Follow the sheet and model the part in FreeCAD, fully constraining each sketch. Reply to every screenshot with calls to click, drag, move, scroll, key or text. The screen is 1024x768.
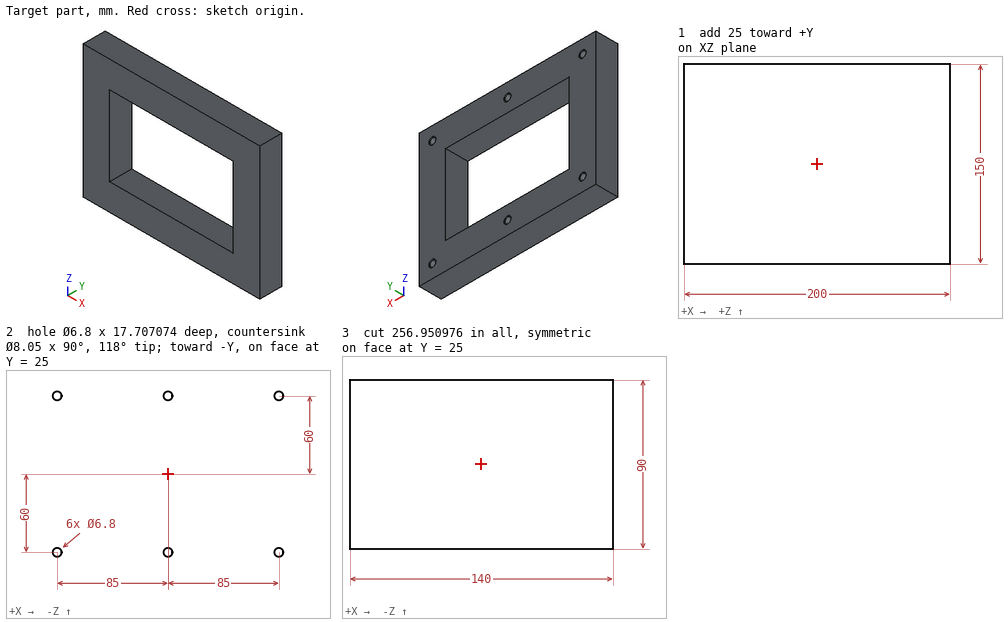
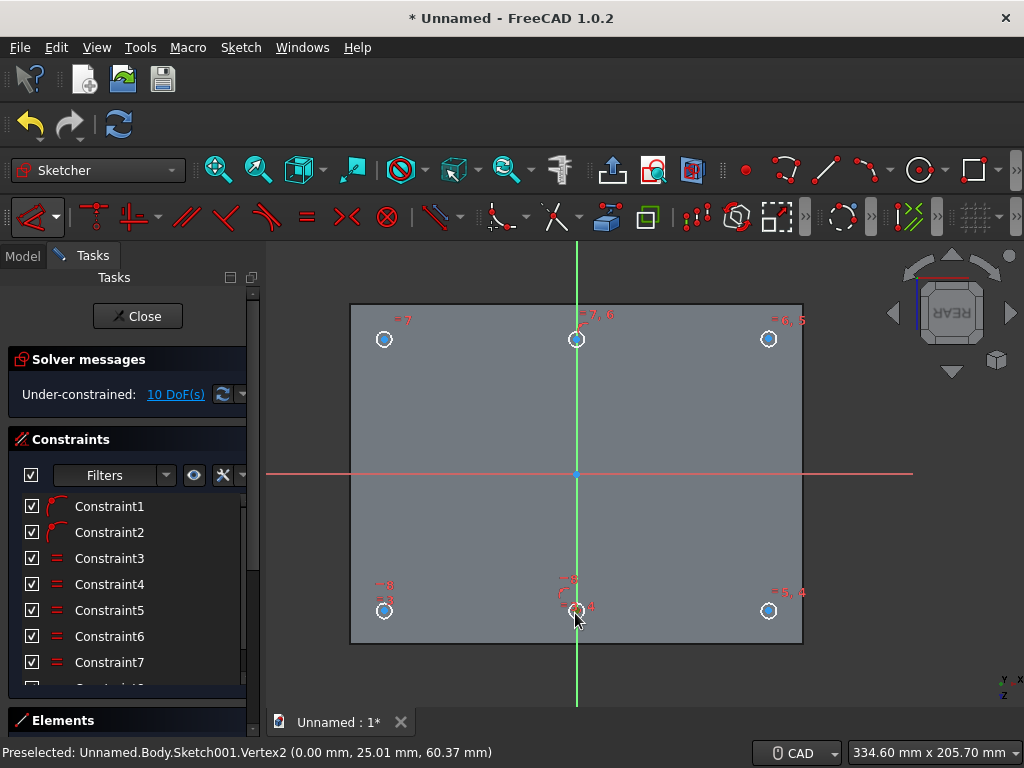
click(769, 611)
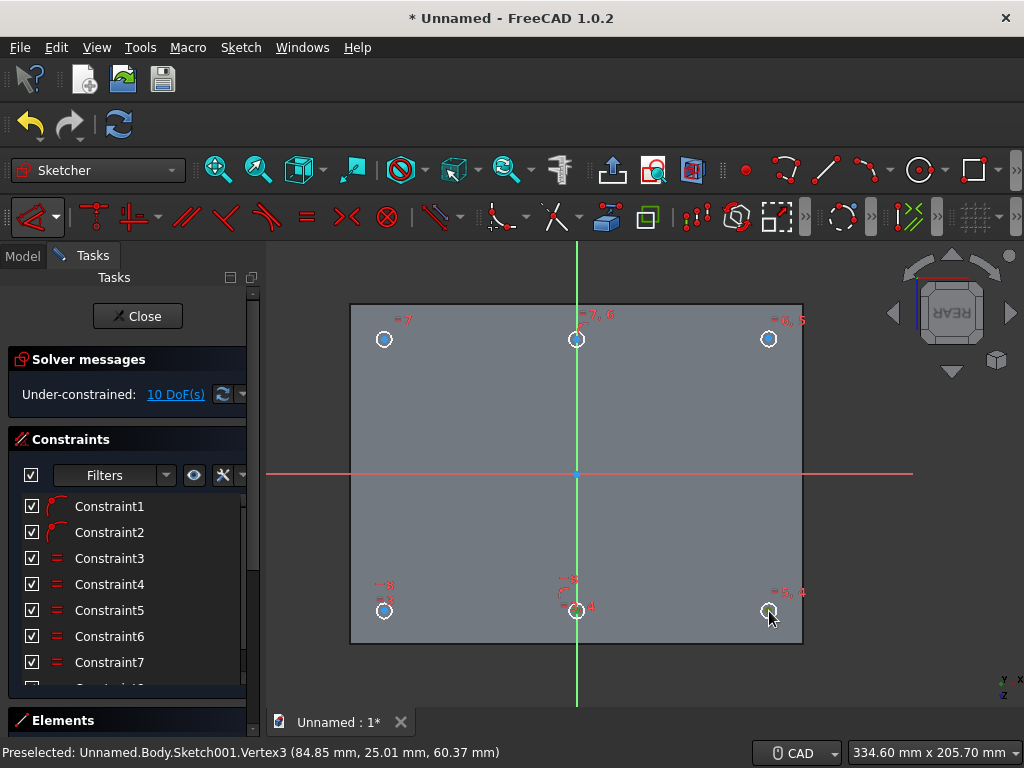
key(h)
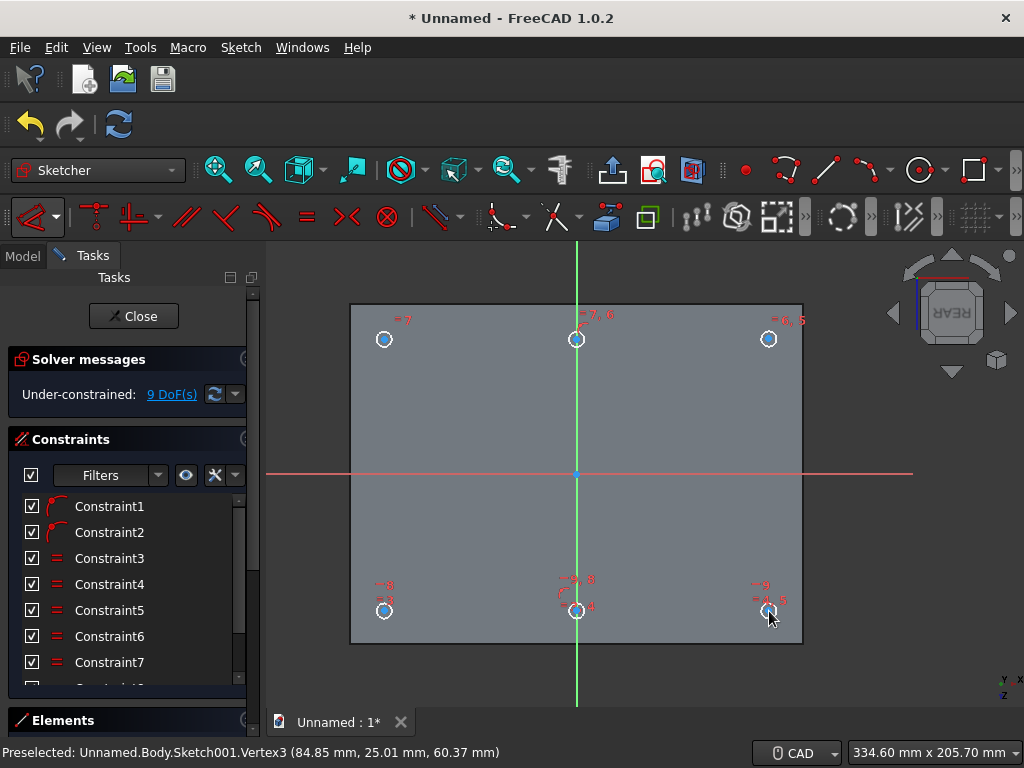
click(769, 611)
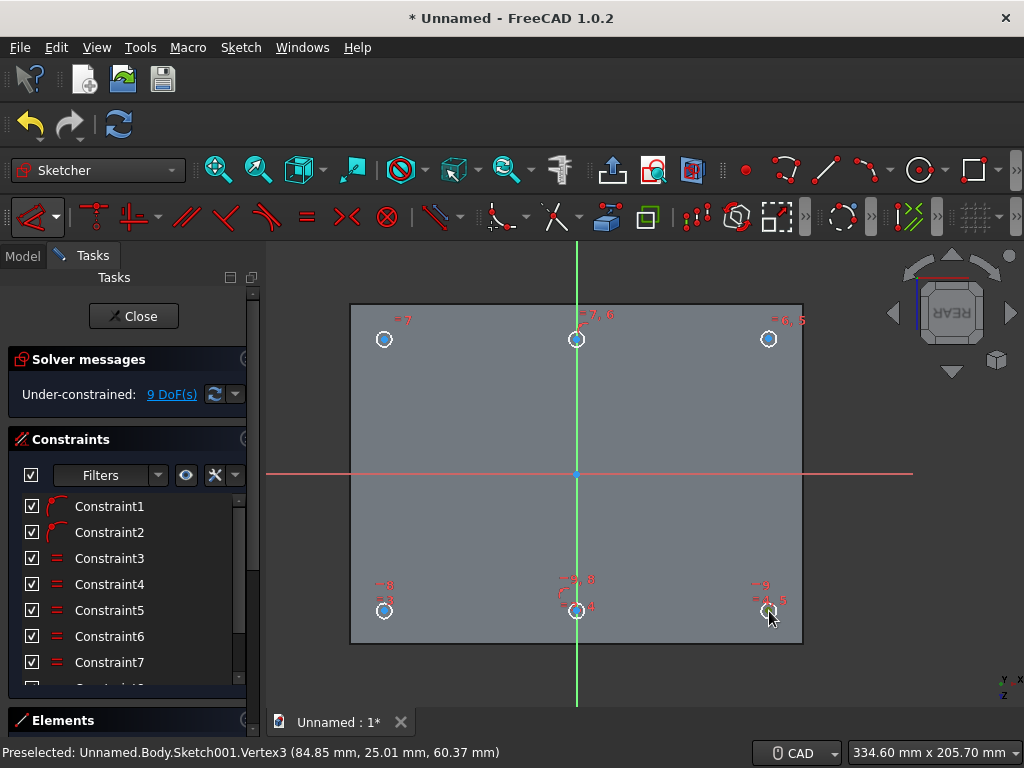
click(769, 339)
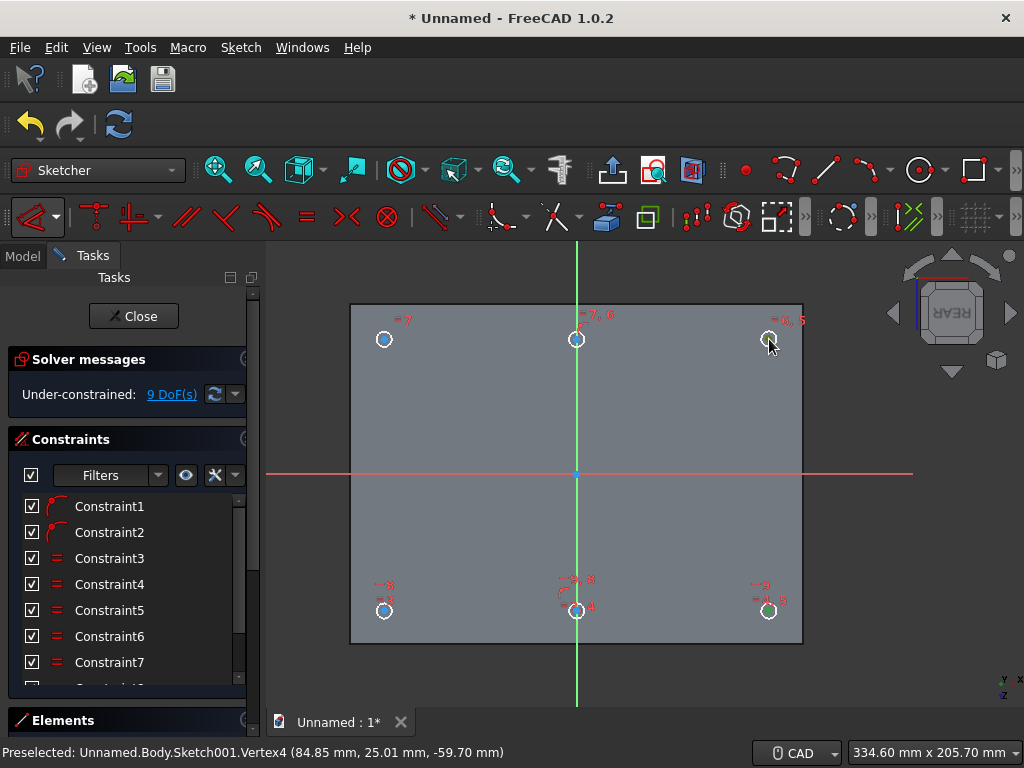
key(v)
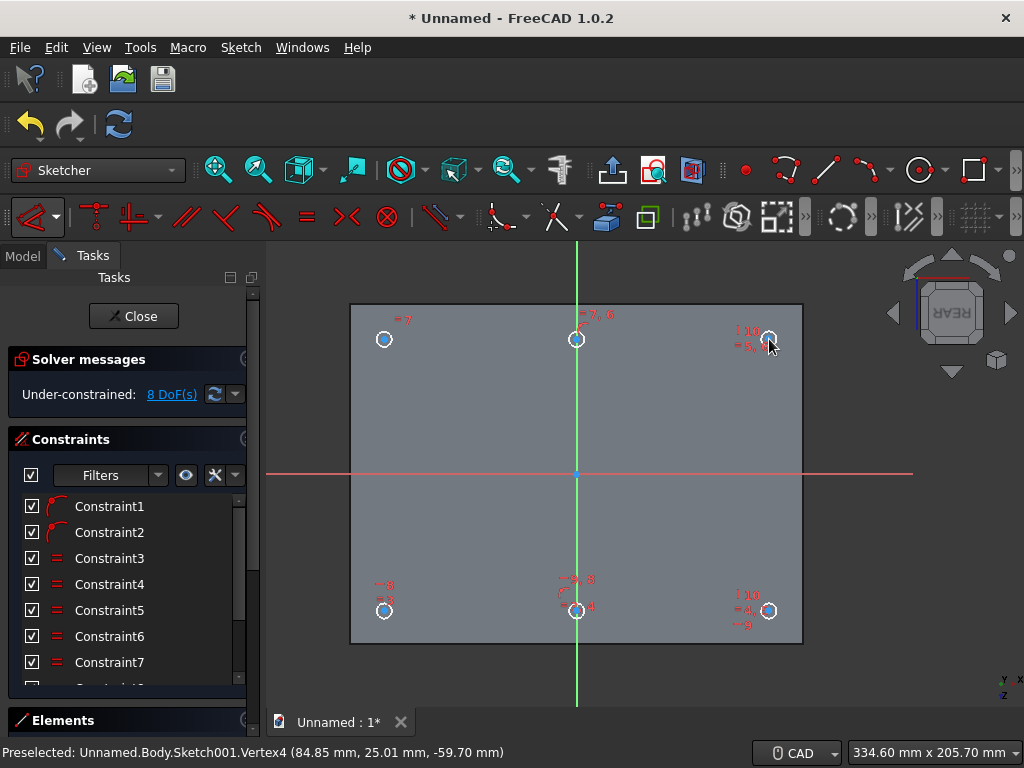
click(769, 339)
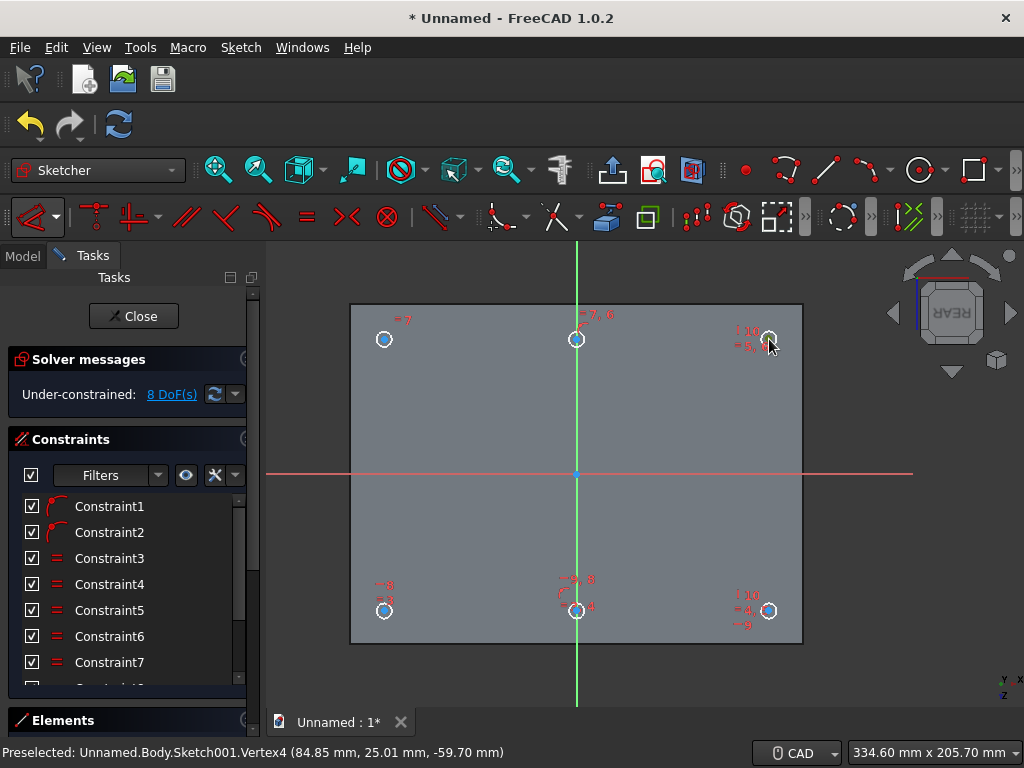
click(577, 339)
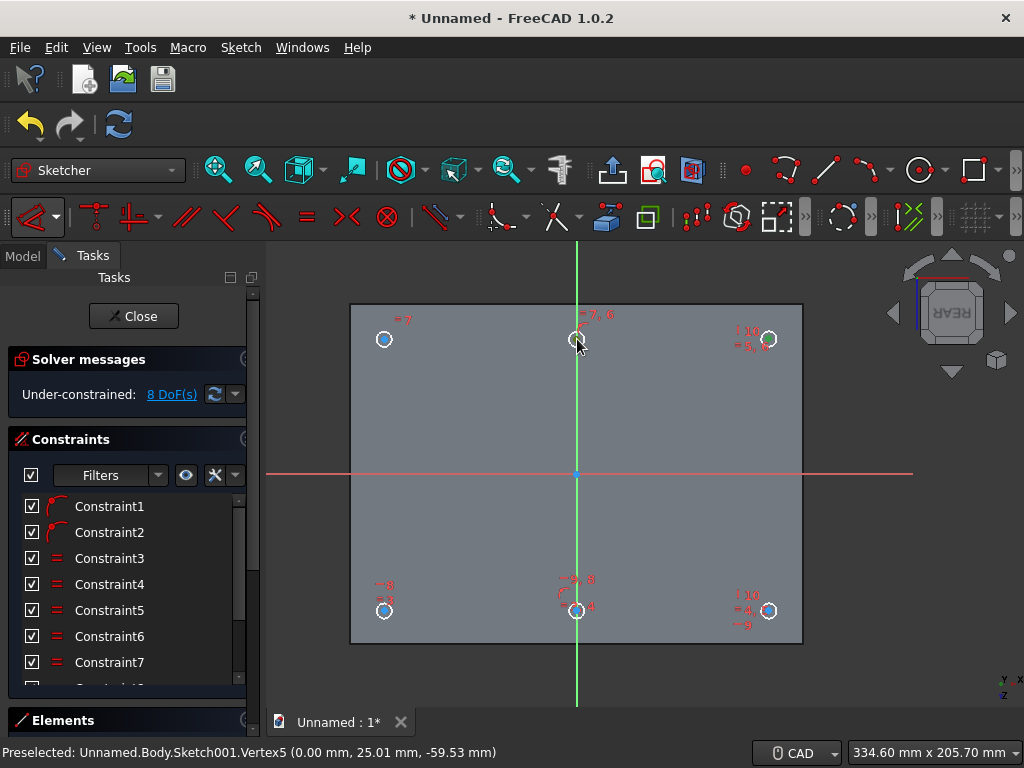
key(h)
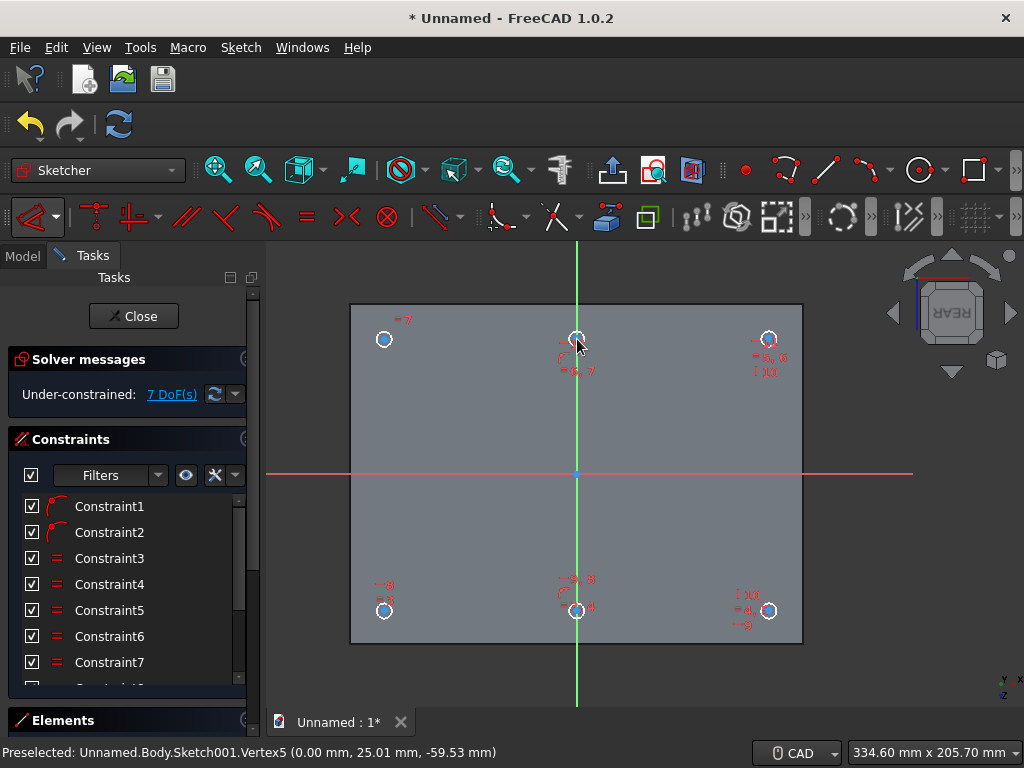
click(384, 611)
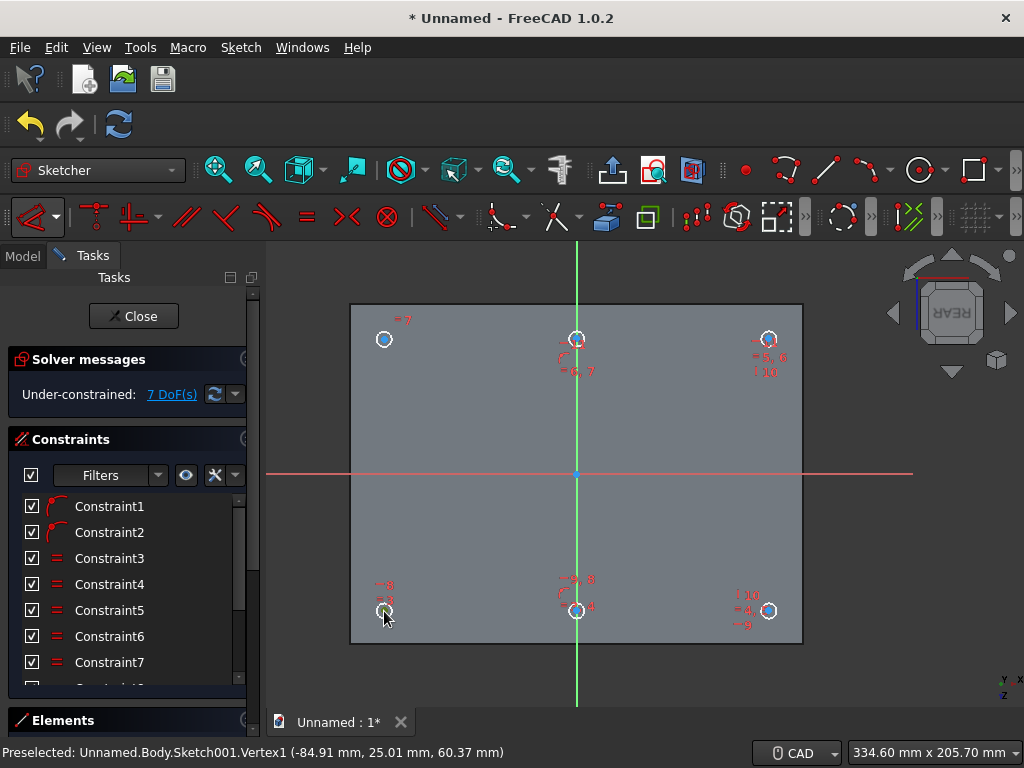
click(384, 339)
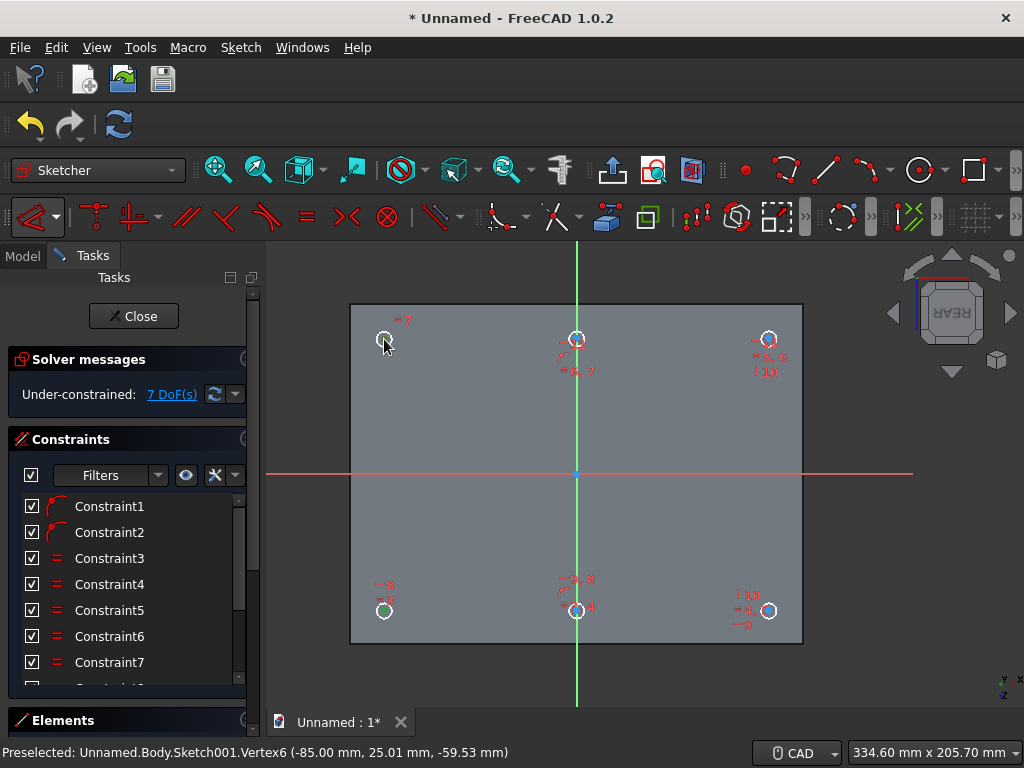
click(160, 218)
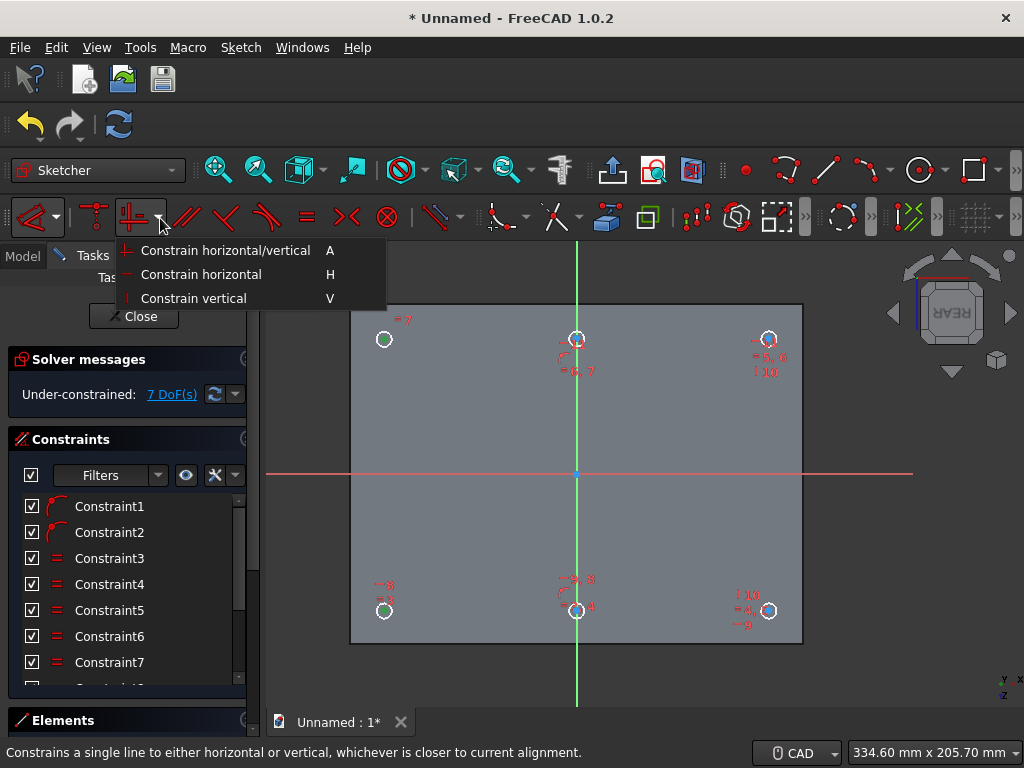
click(251, 298)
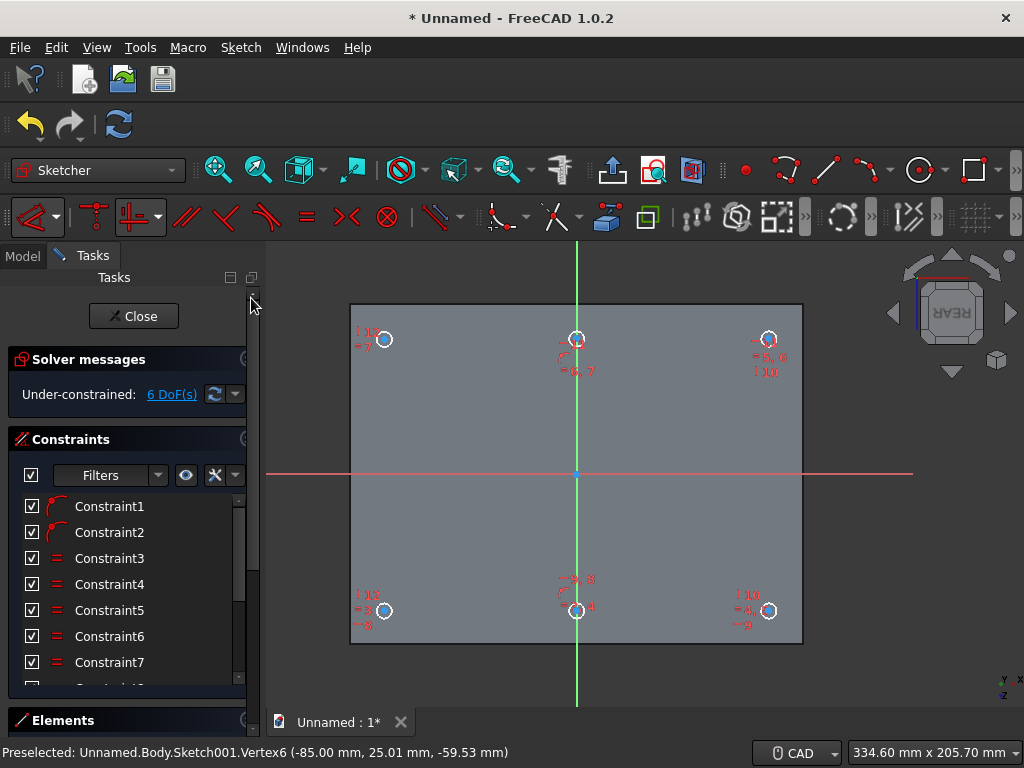
scroll(577, 339, up, 4)